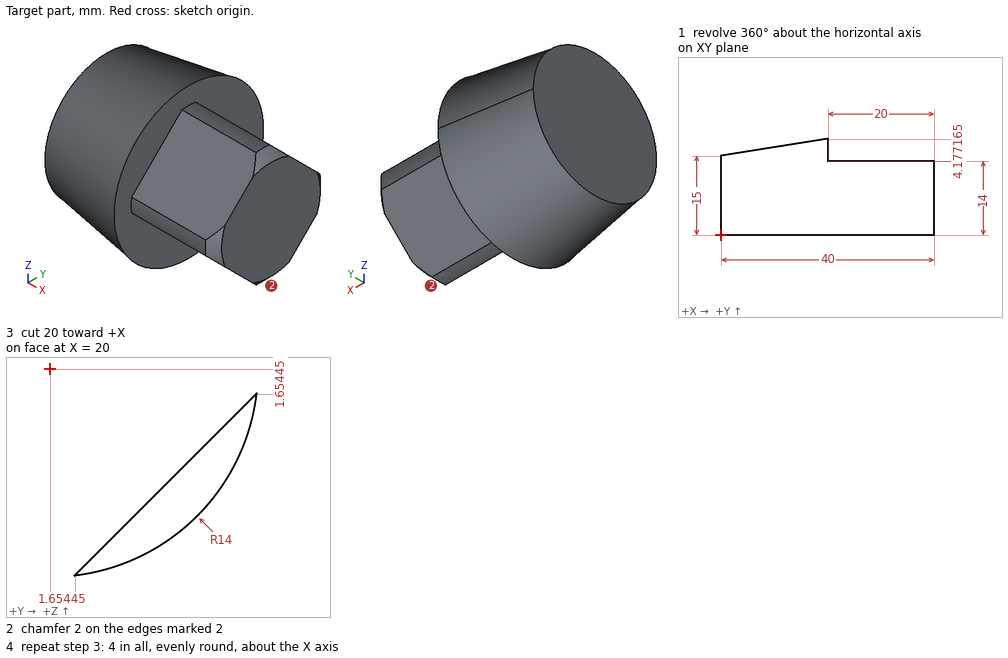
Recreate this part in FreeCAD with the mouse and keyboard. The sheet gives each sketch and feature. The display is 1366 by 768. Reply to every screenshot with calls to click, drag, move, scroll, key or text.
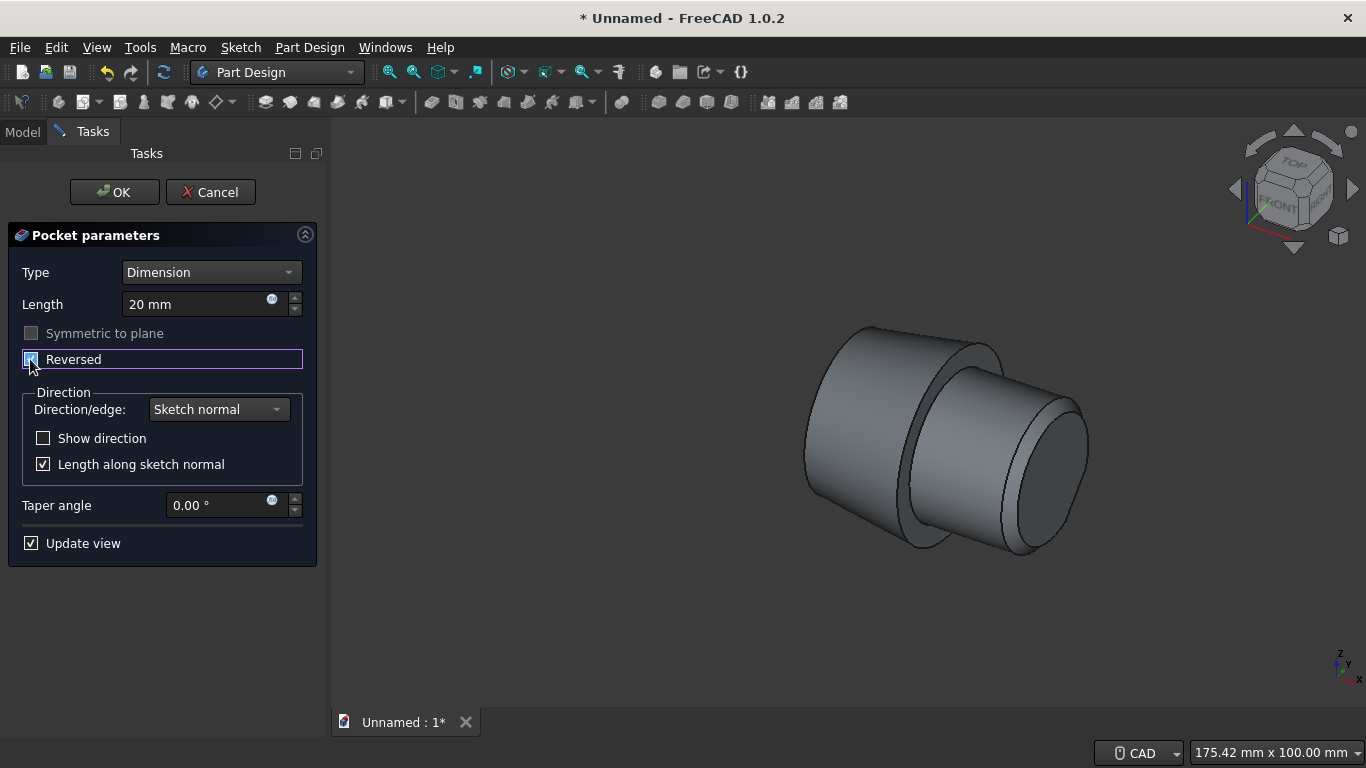
click(115, 192)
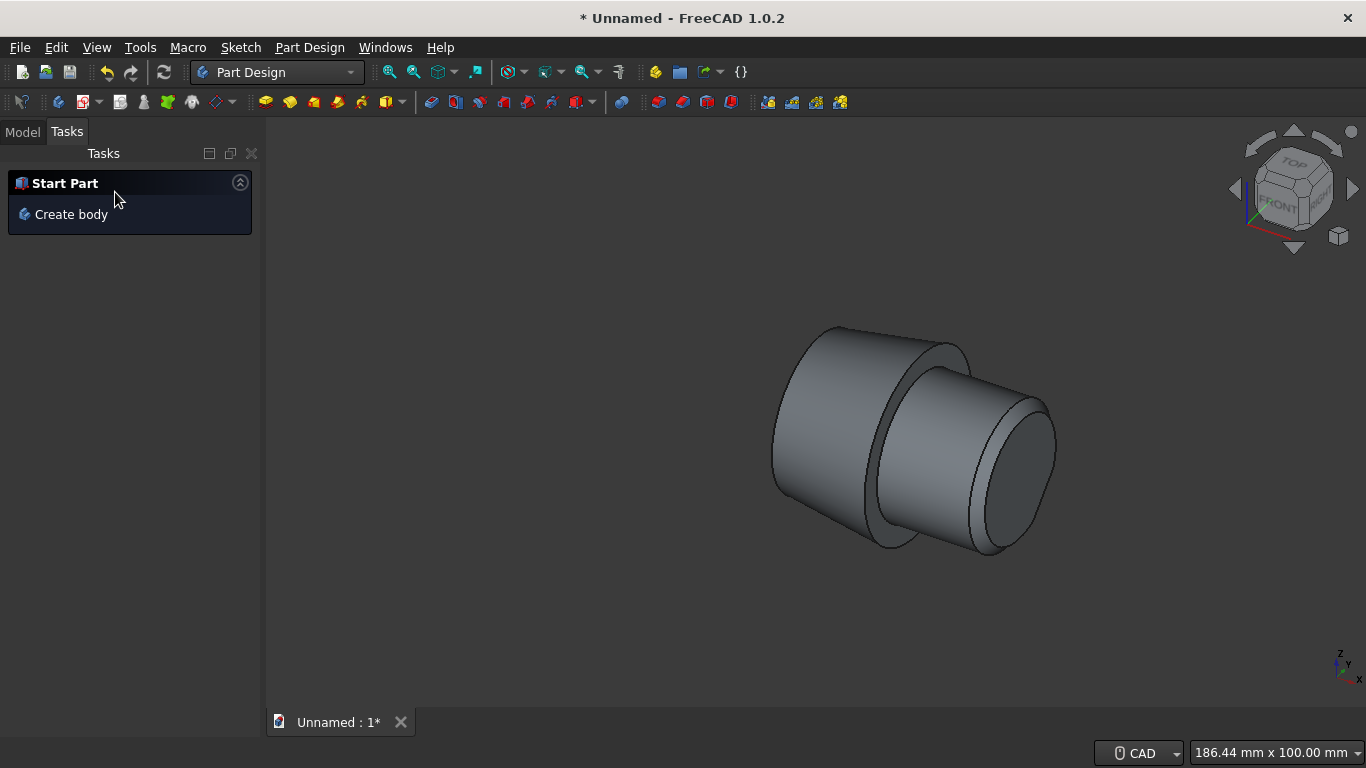
click(23, 131)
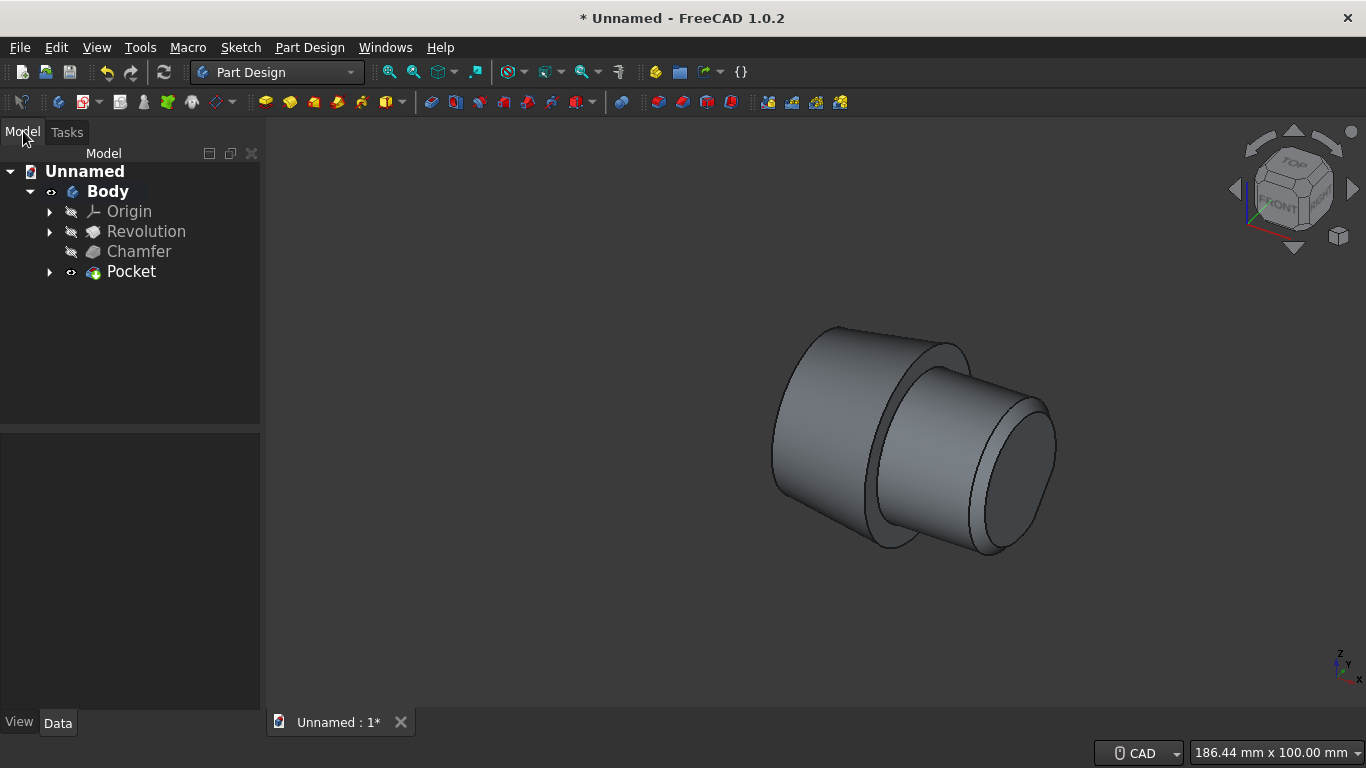
click(116, 272)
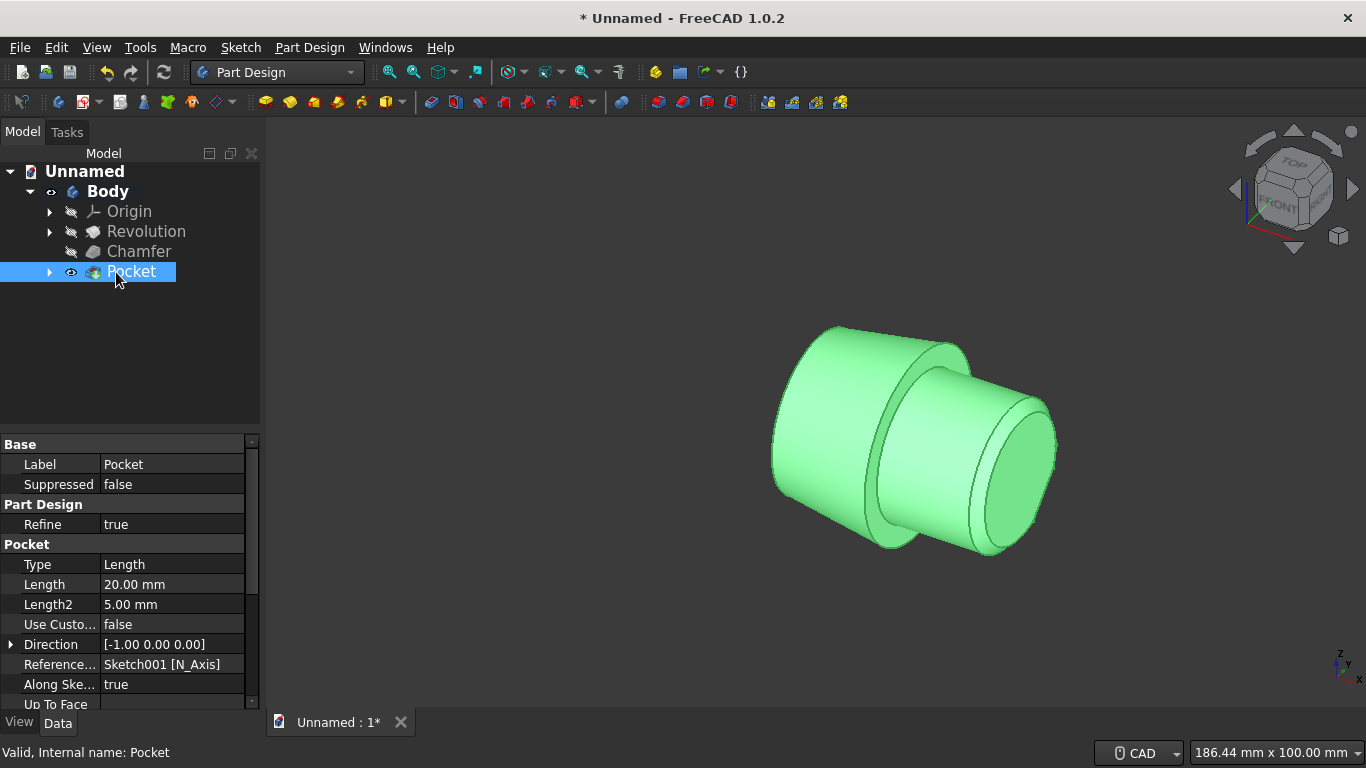
click(816, 102)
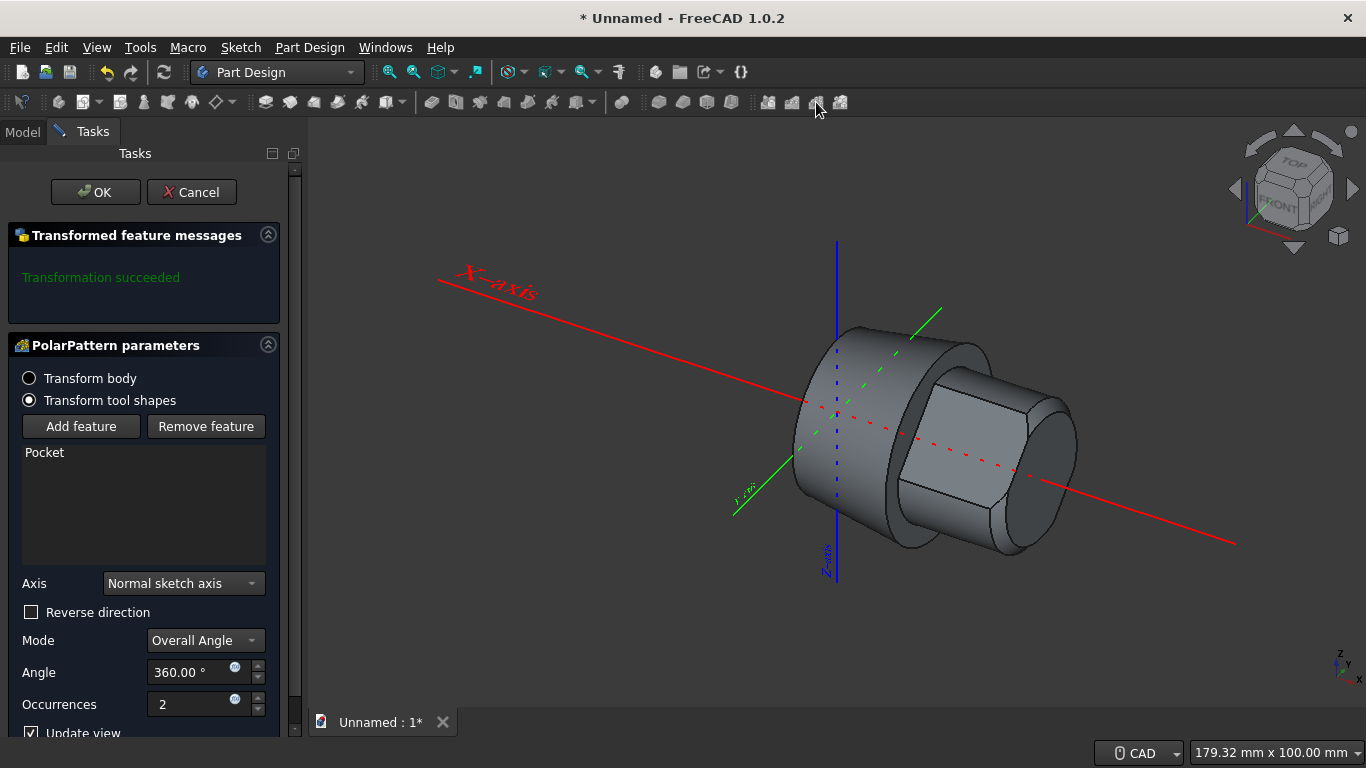
click(184, 584)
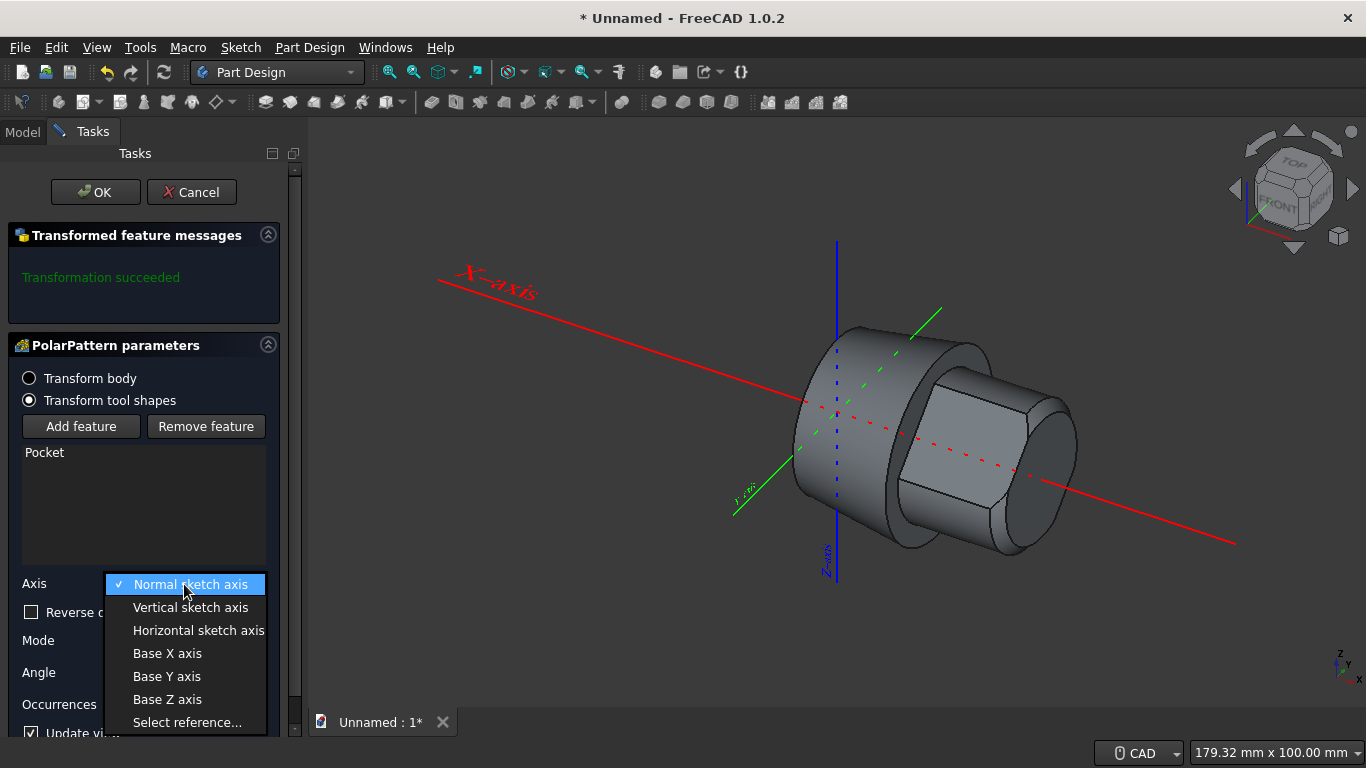
click(184, 654)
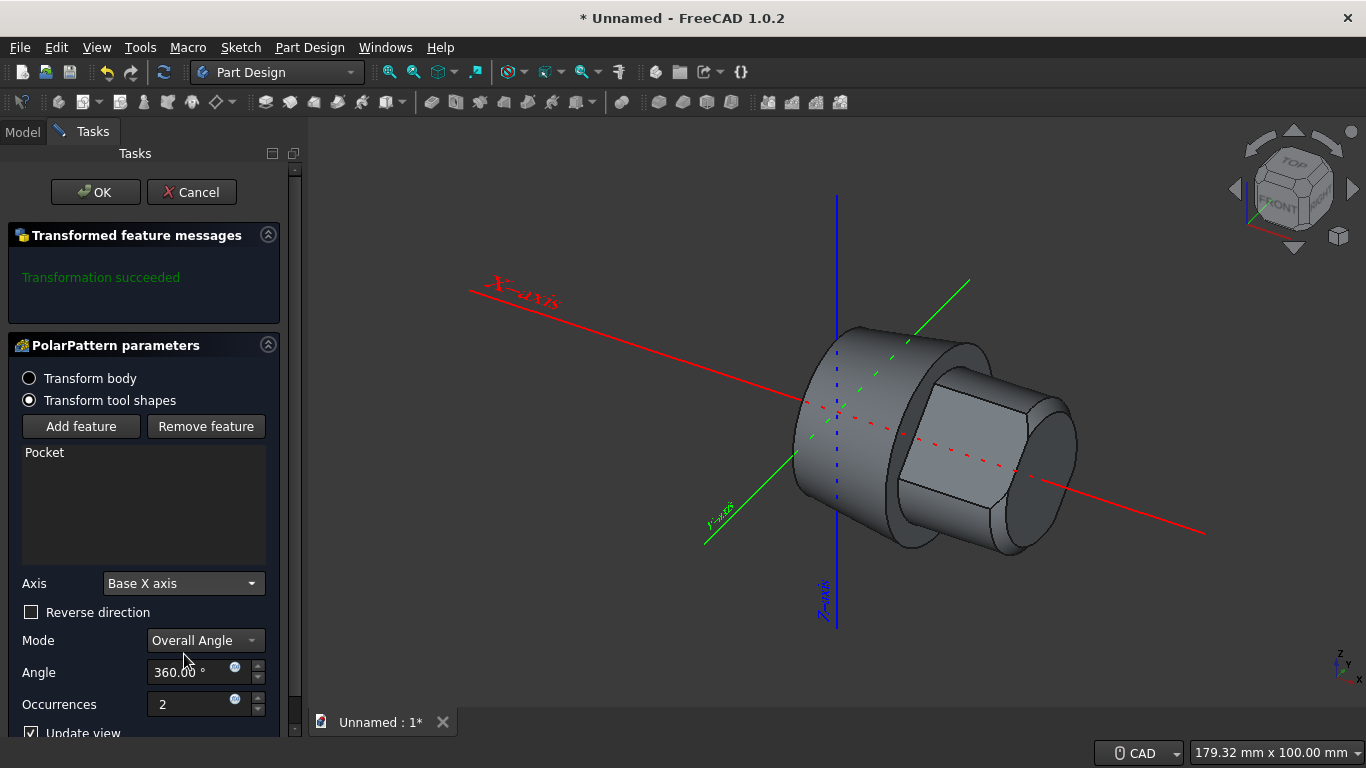
triple_click(198, 704)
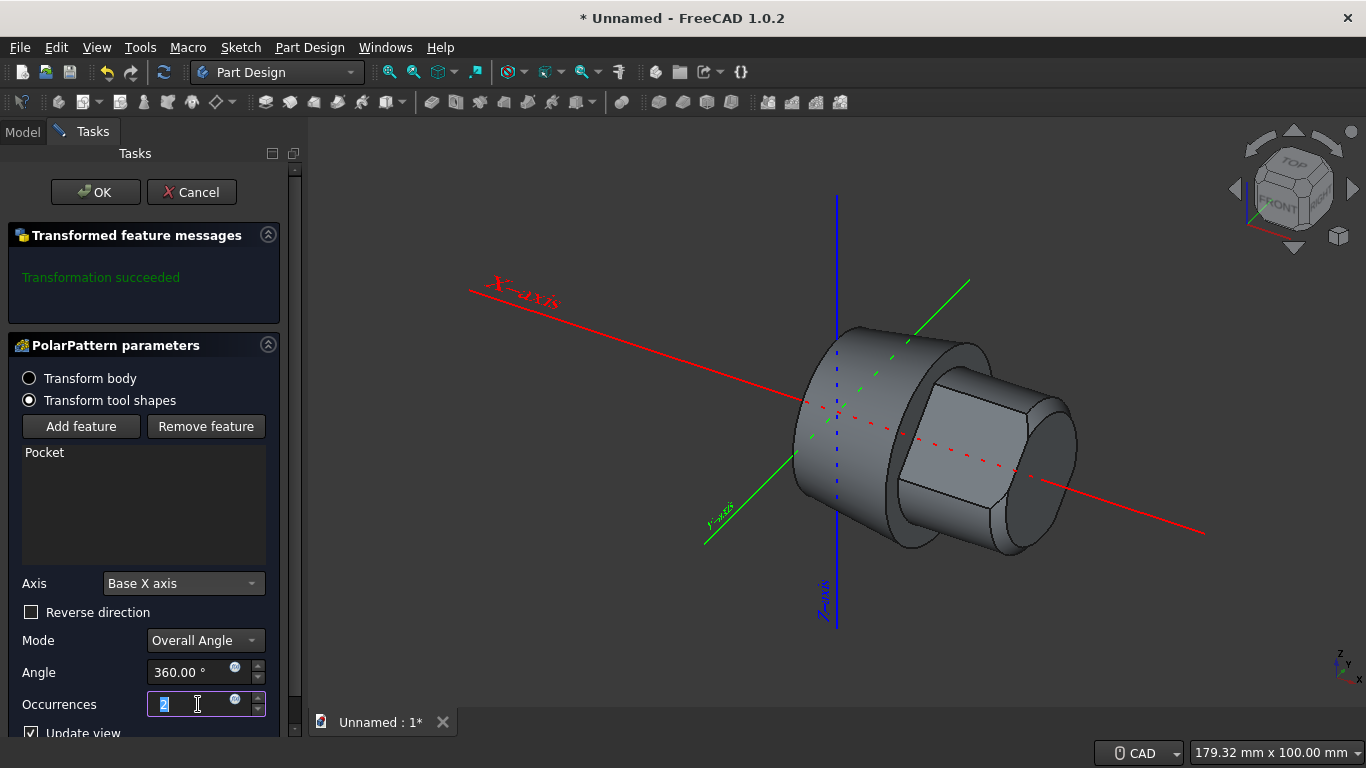
text(4)
key(Tab)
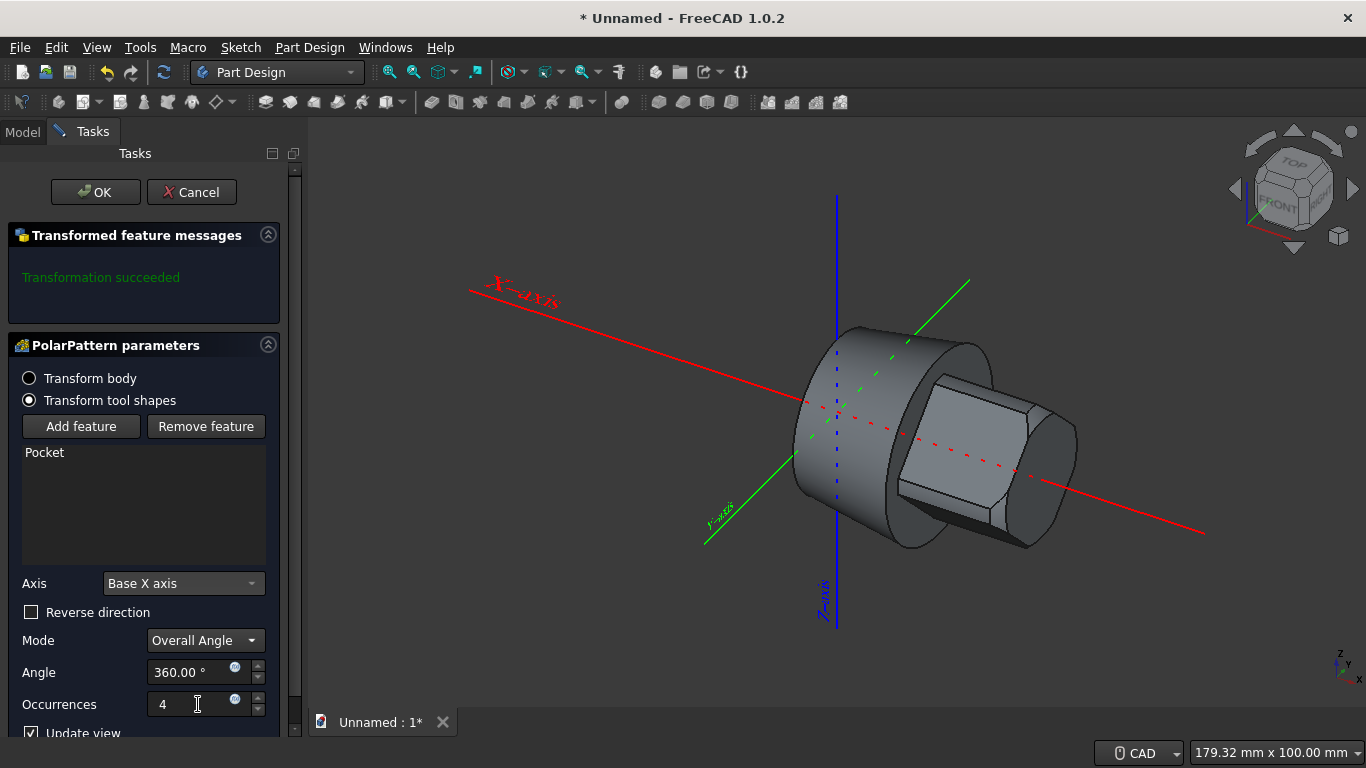
click(96, 192)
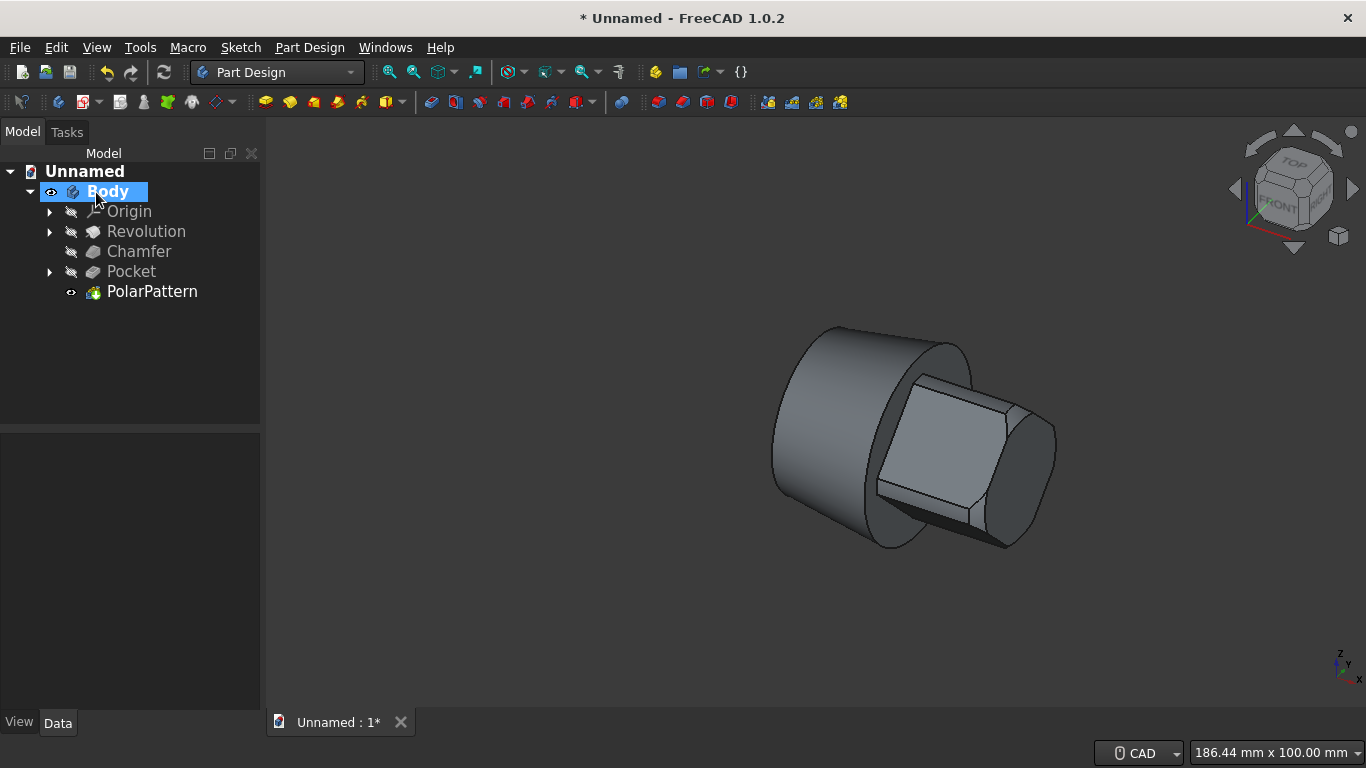
key(0)